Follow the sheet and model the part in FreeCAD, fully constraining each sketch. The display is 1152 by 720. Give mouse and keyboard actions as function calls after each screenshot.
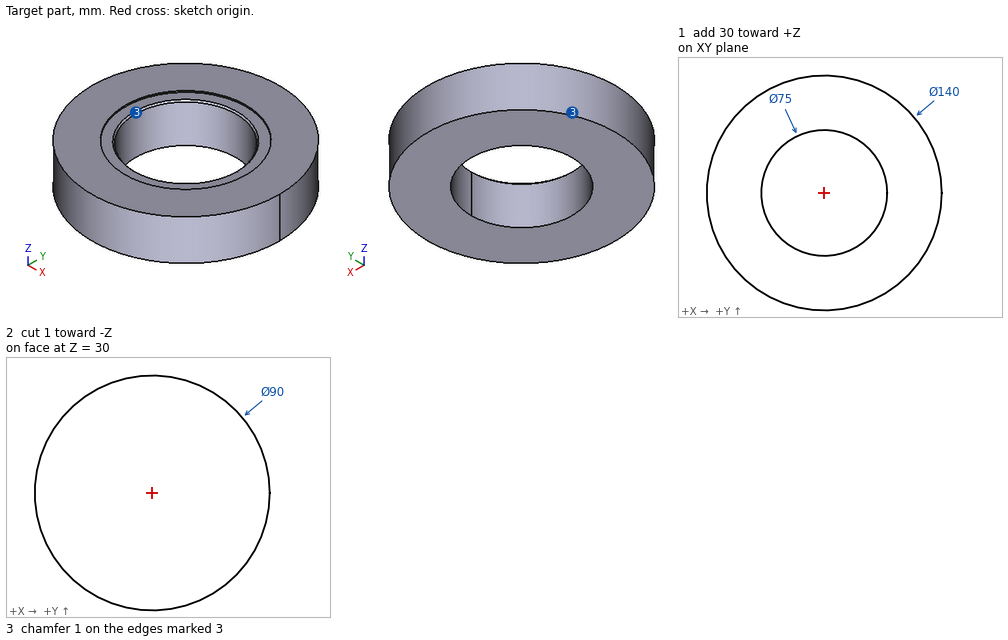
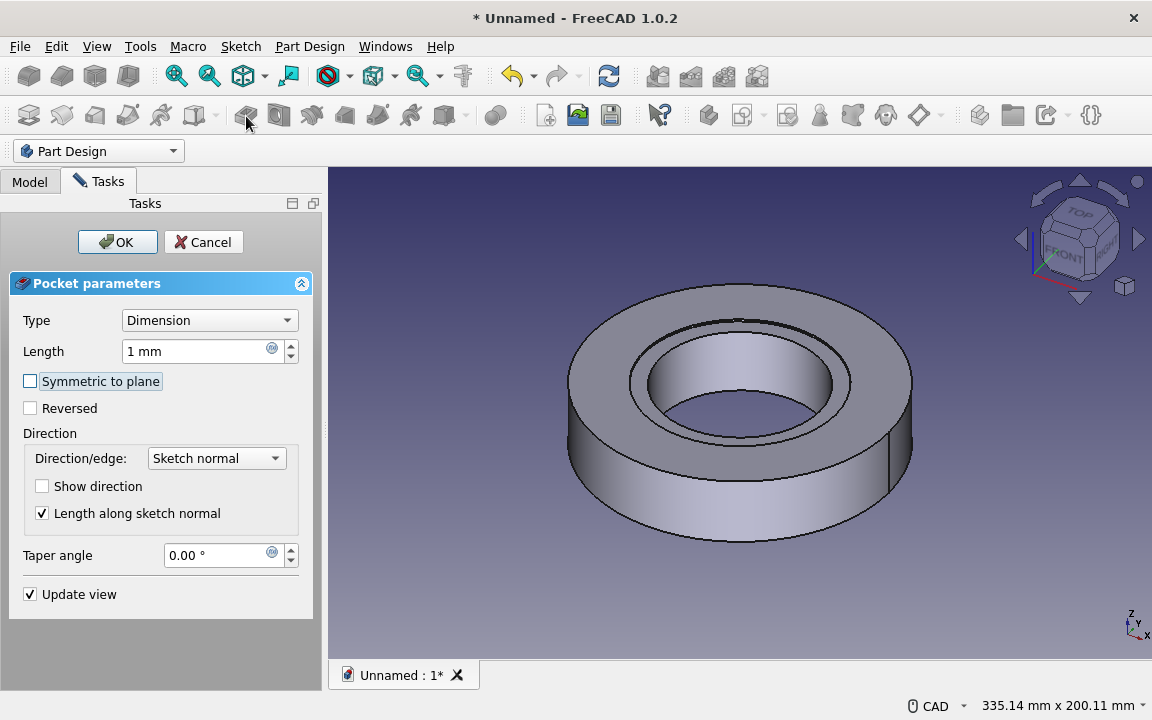
click(118, 242)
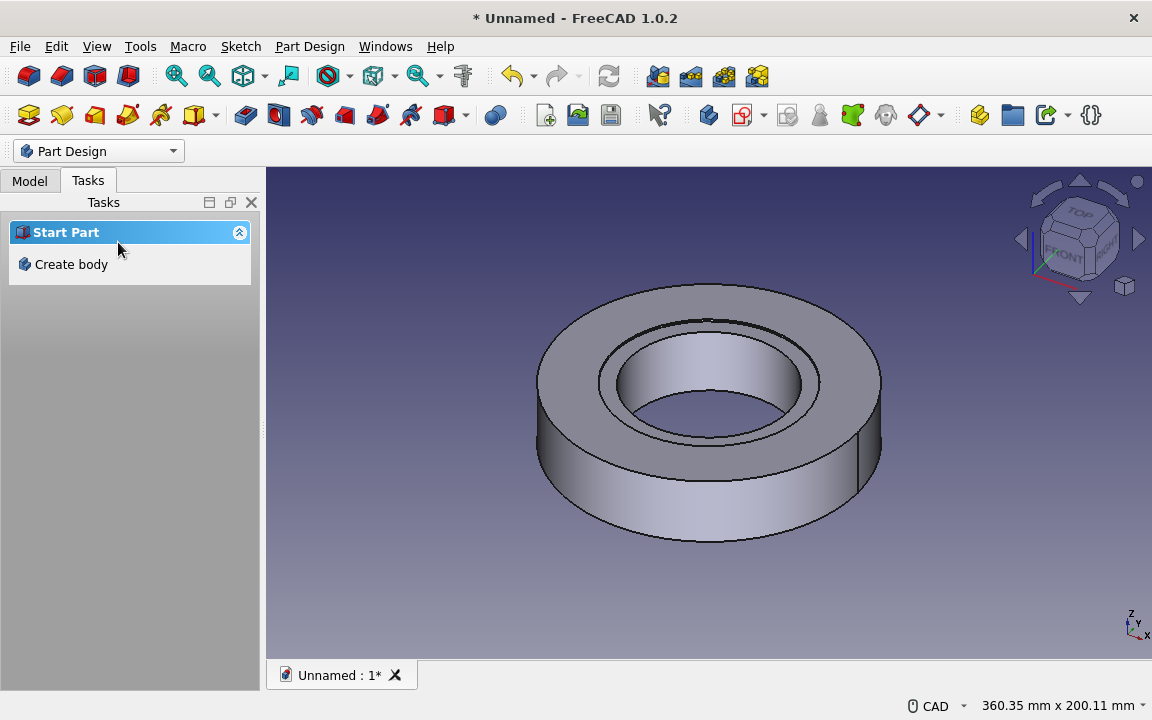
click(629, 357)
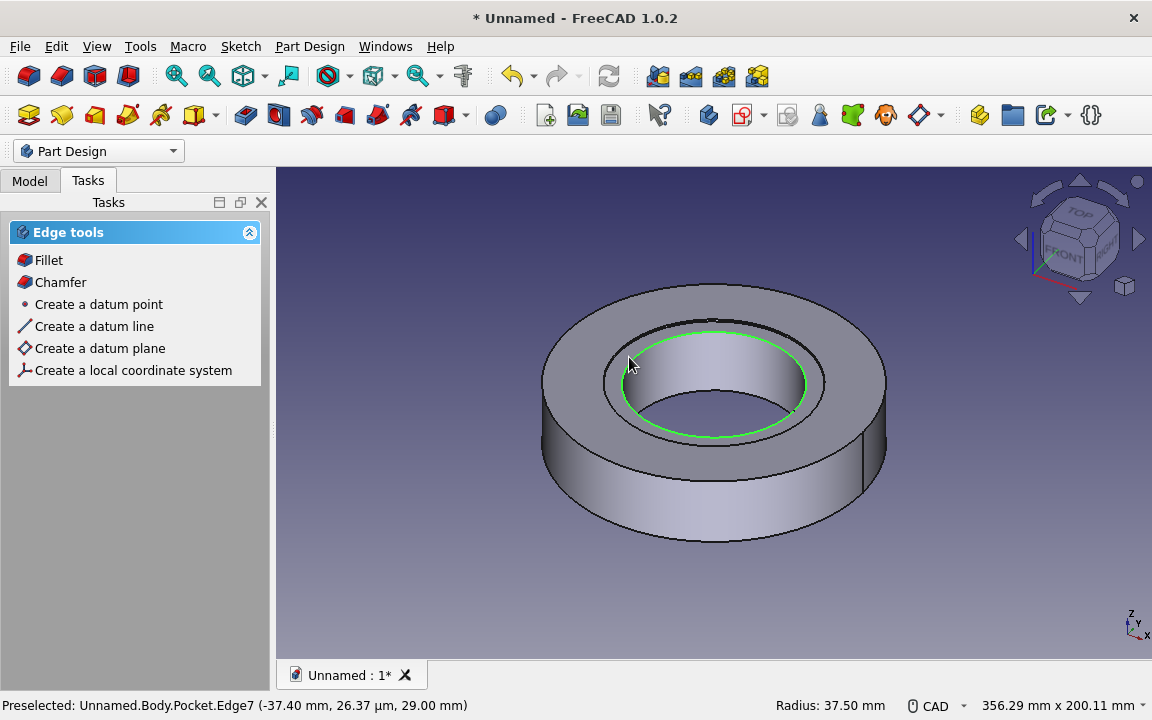
click(62, 76)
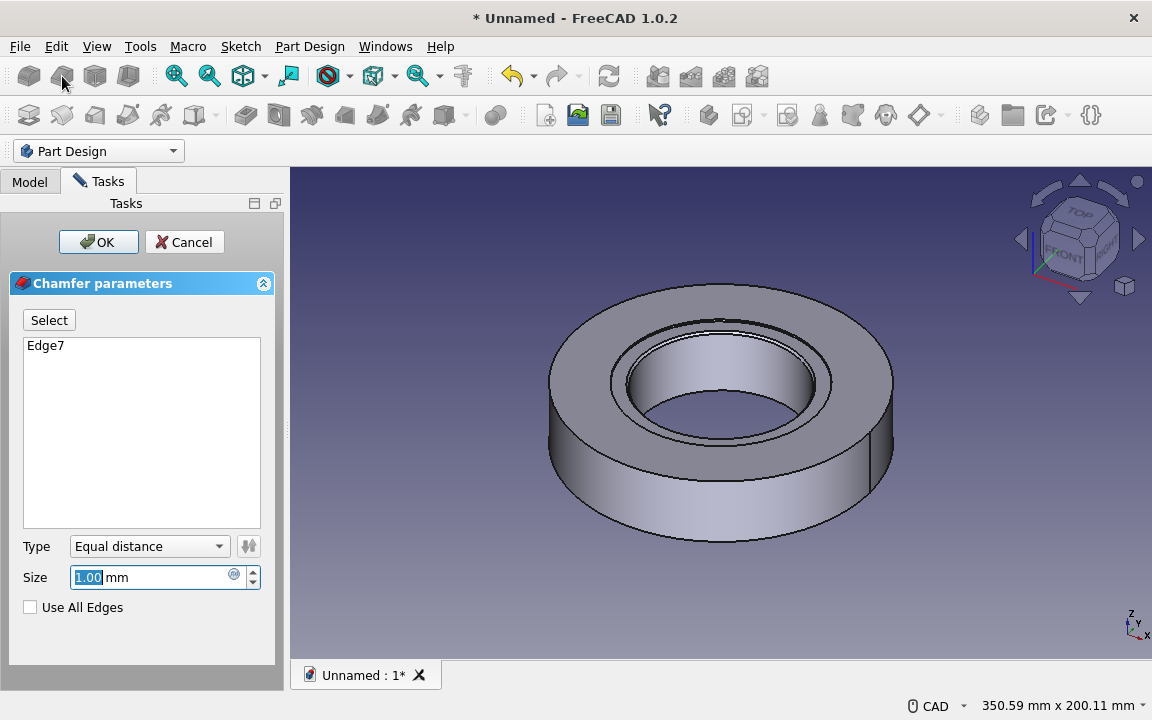
text(1)
key(Tab)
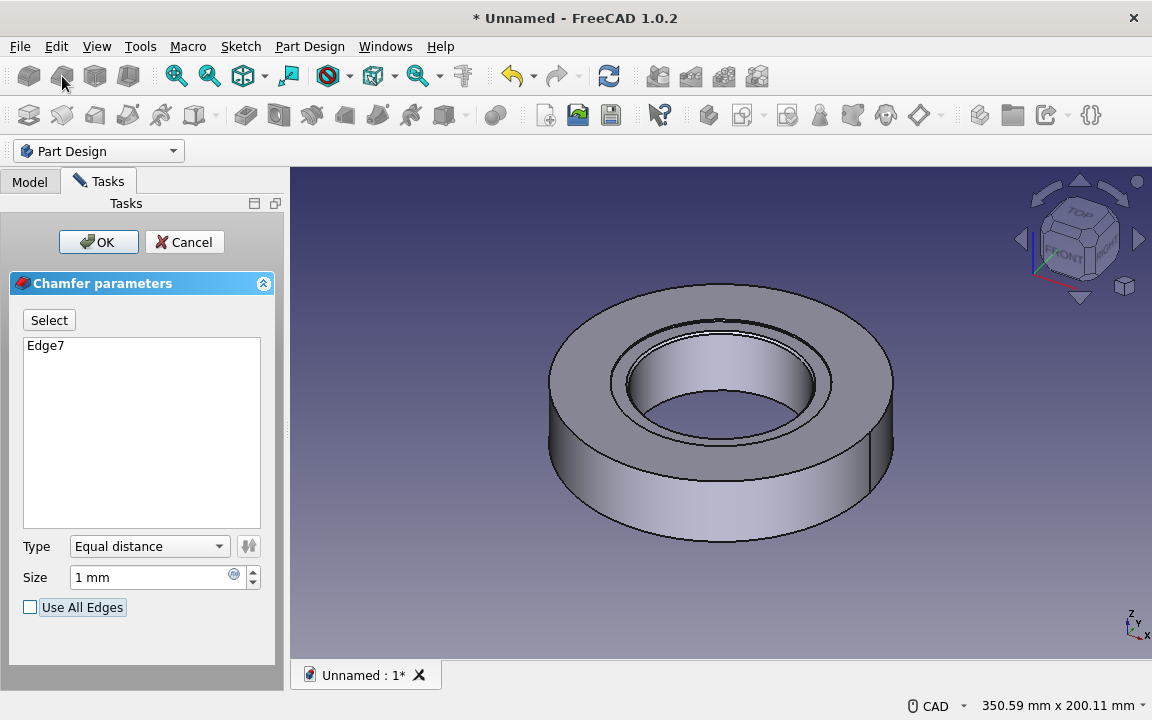
click(99, 242)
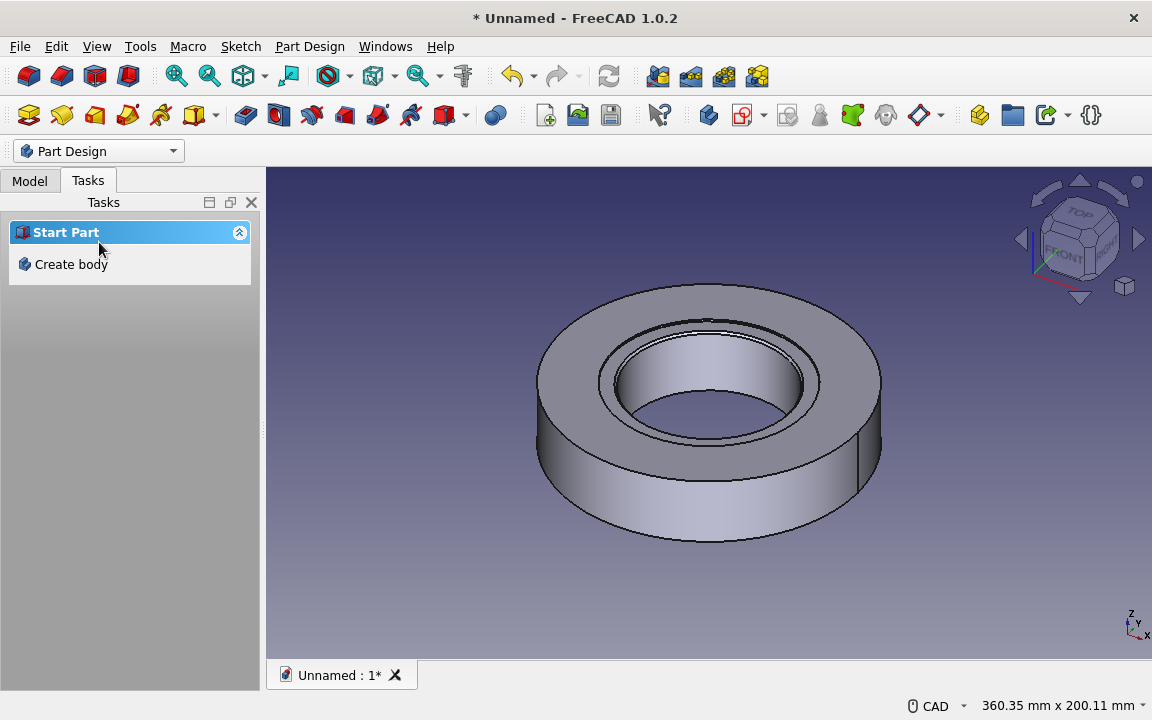
key(0)